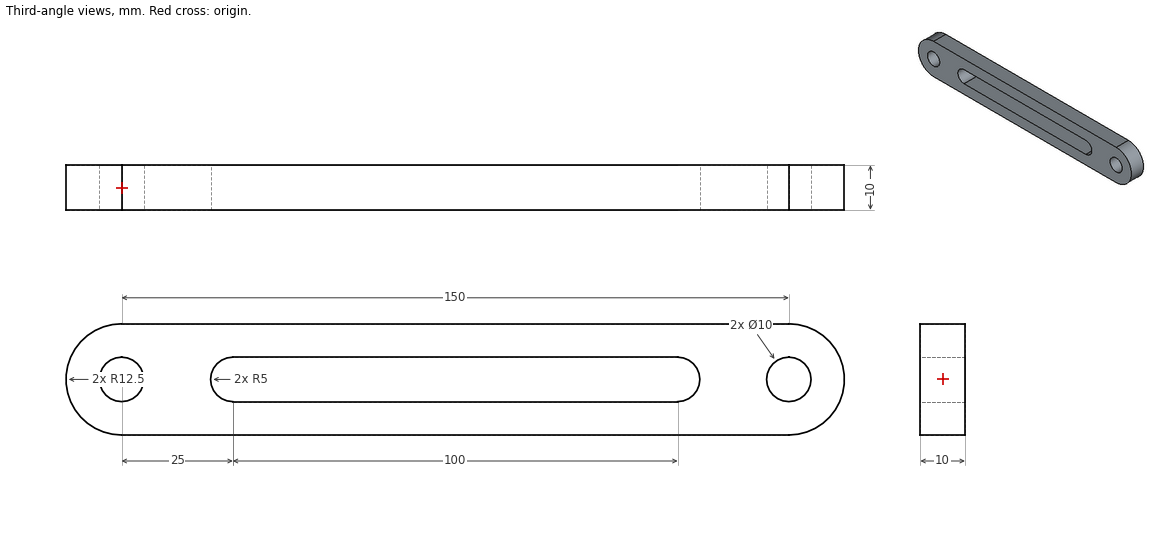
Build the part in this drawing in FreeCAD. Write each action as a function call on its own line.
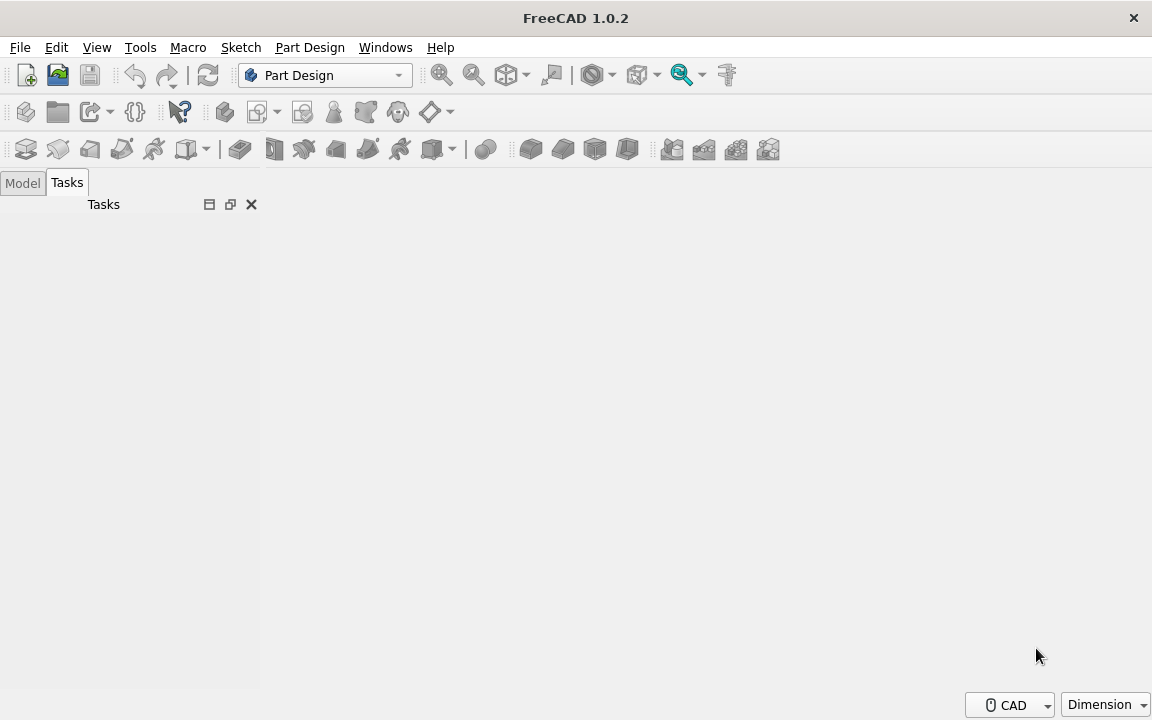
click(510, 112)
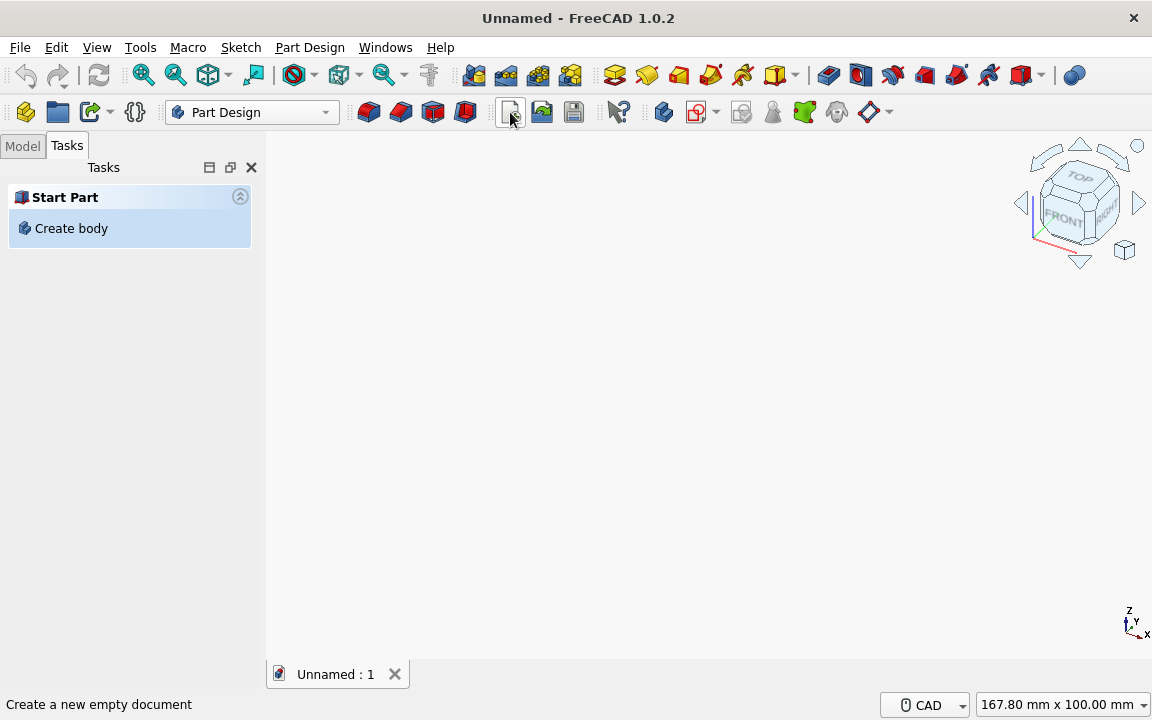
click(696, 112)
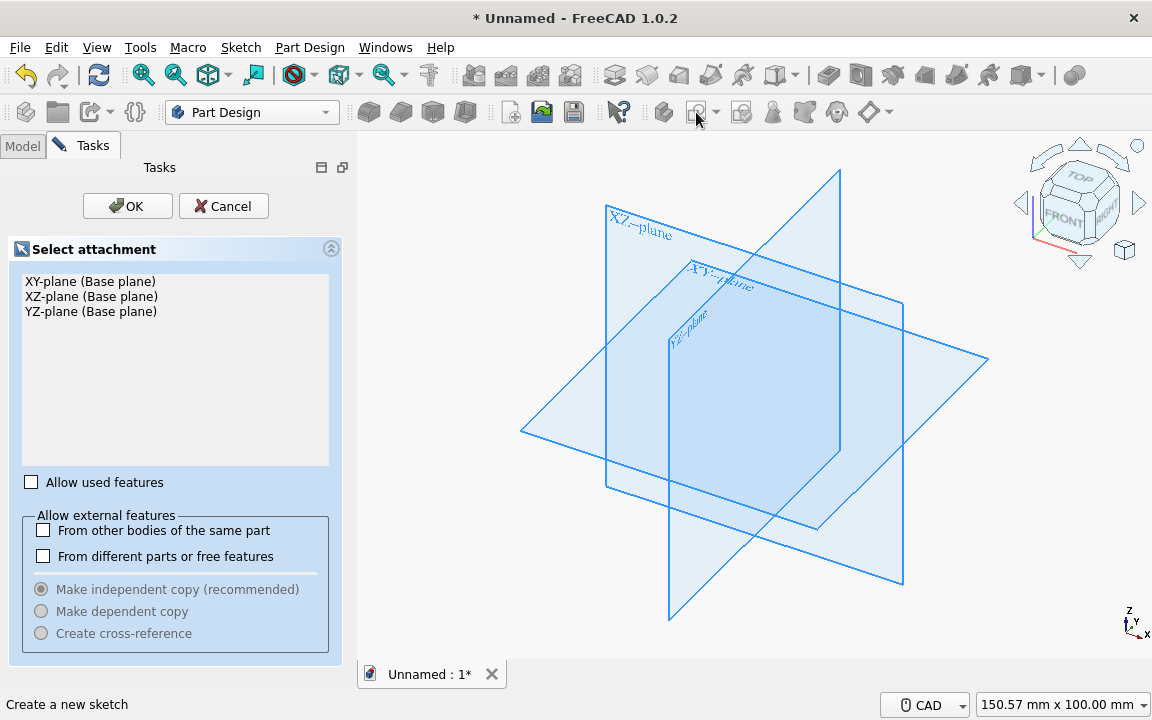
click(82, 296)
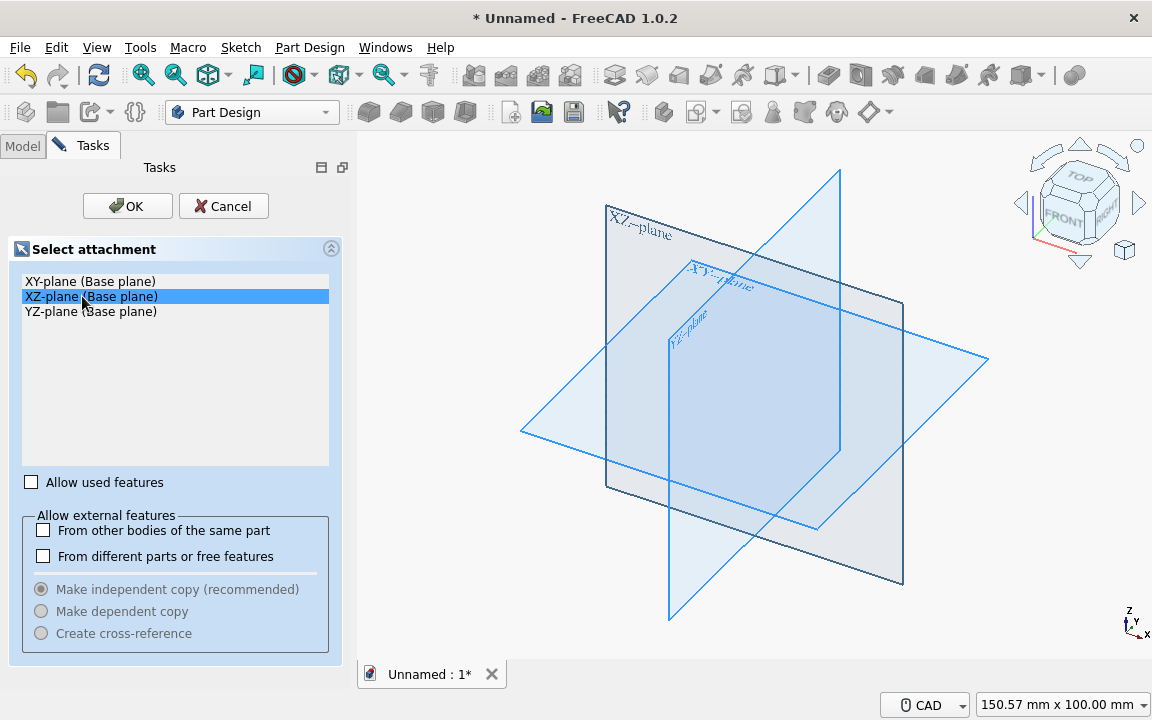
click(128, 206)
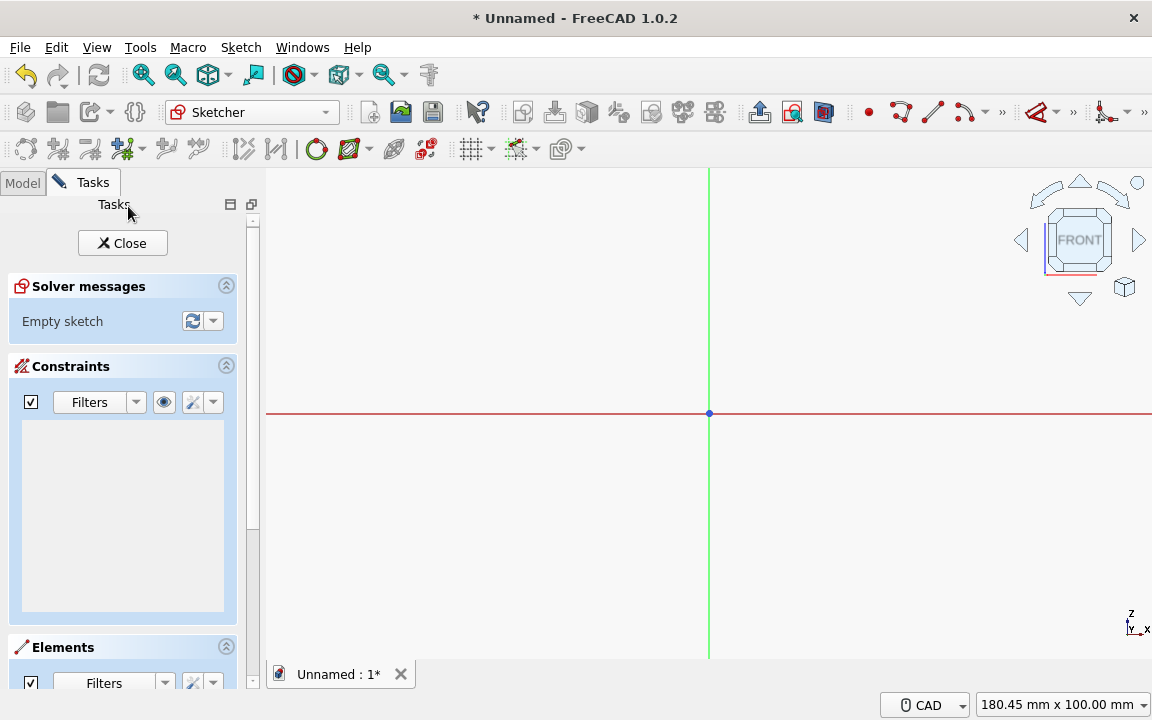
scroll(294, 414, down, 3)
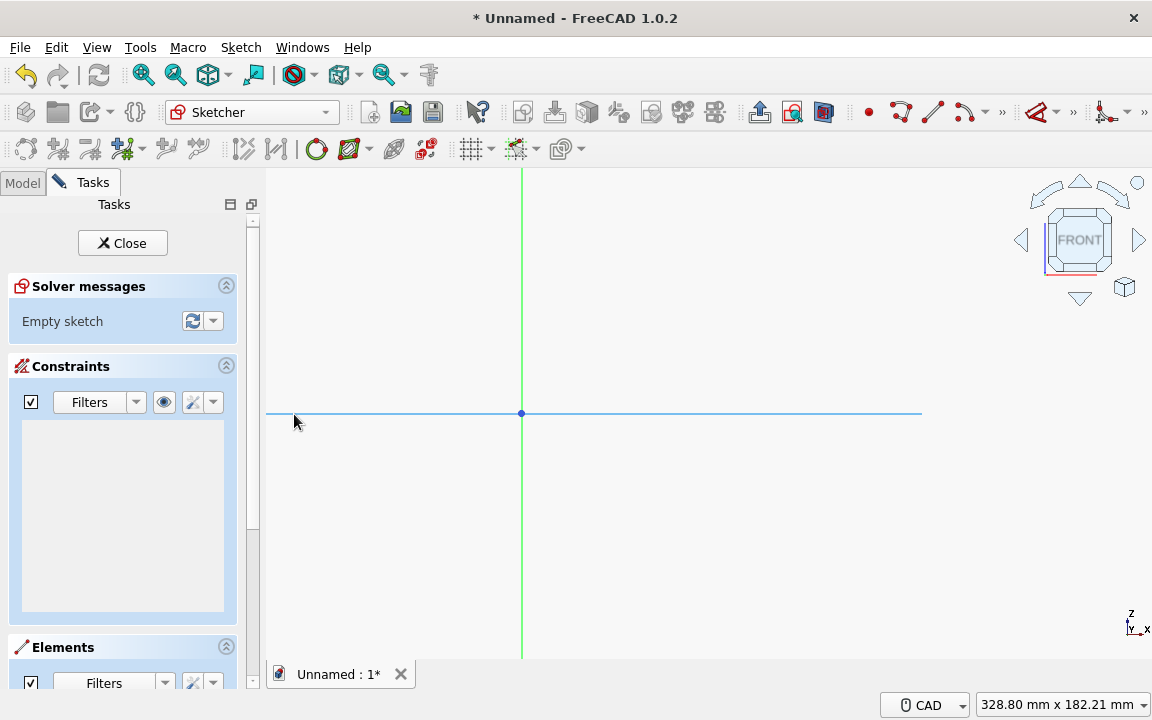
key(g)
key(s)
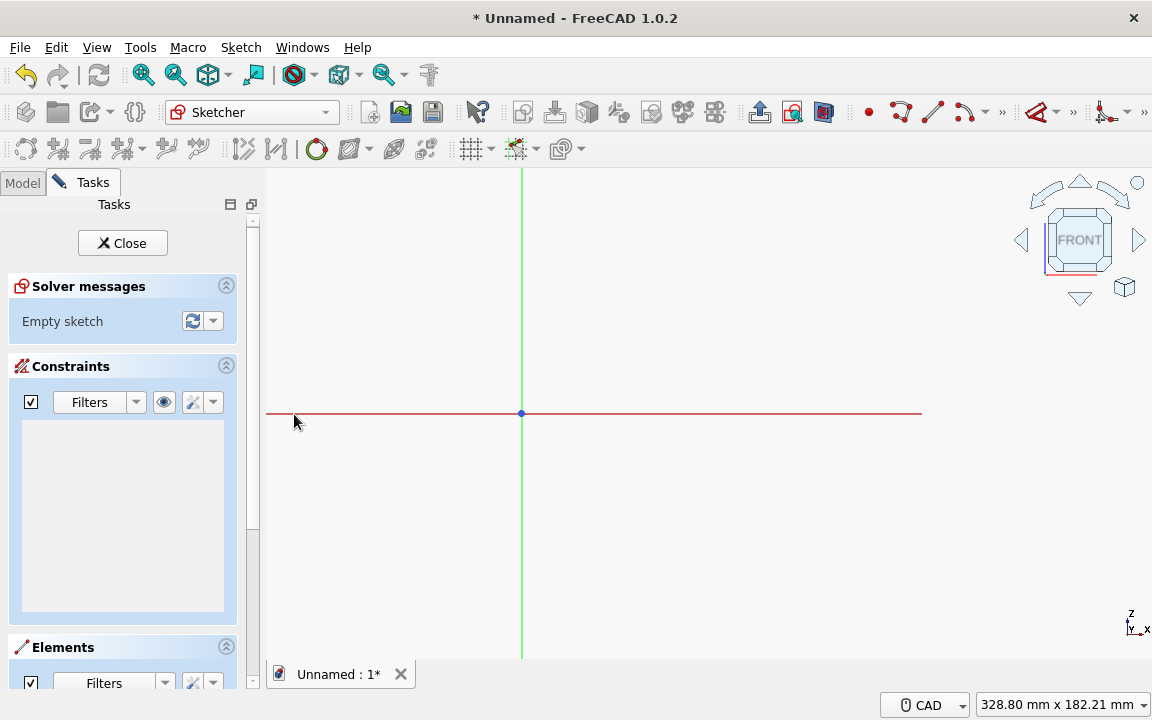
click(522, 414)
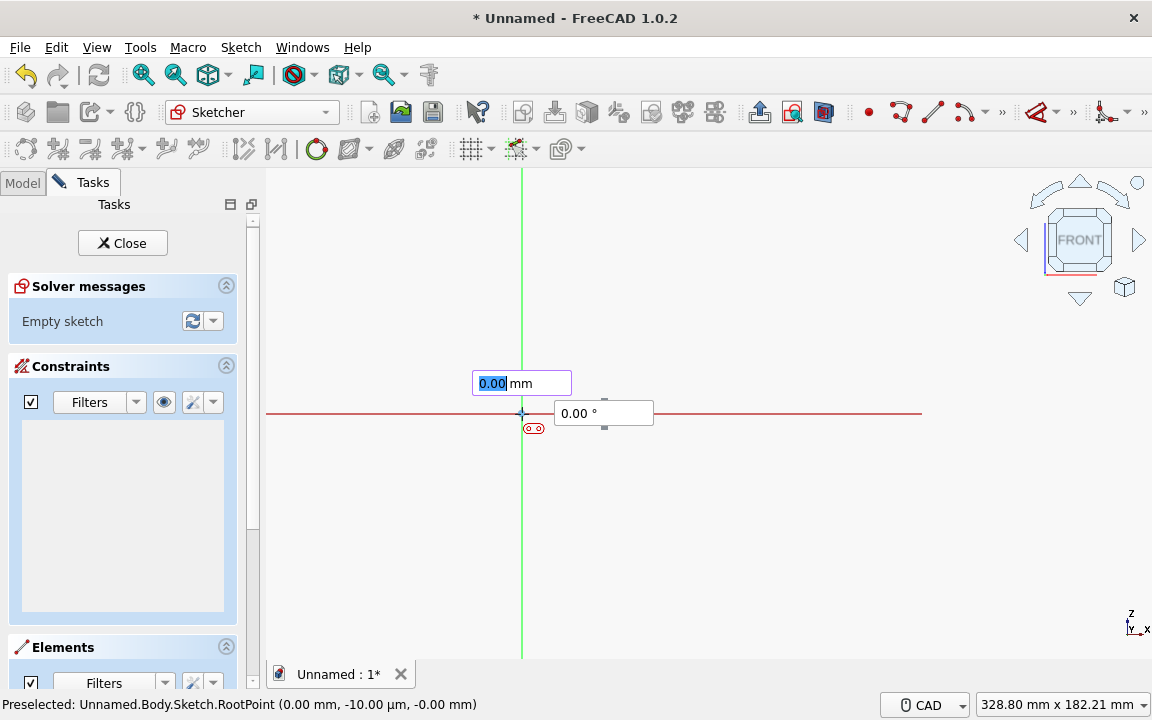
click(926, 405)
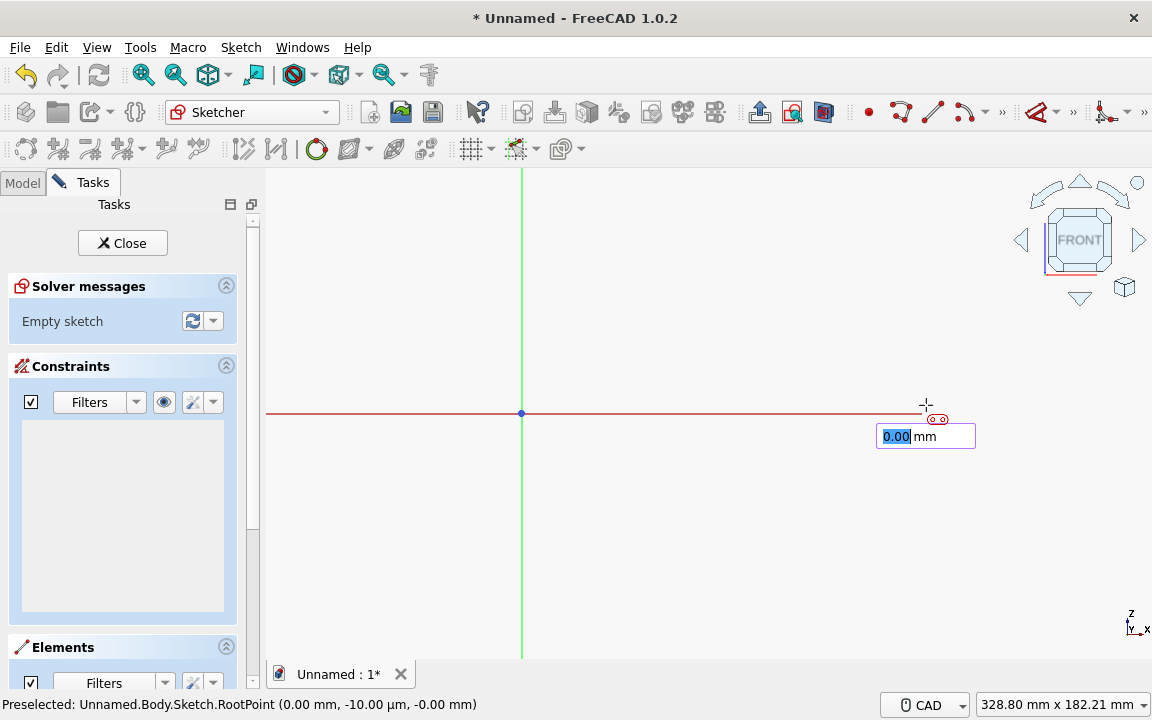
click(724, 448)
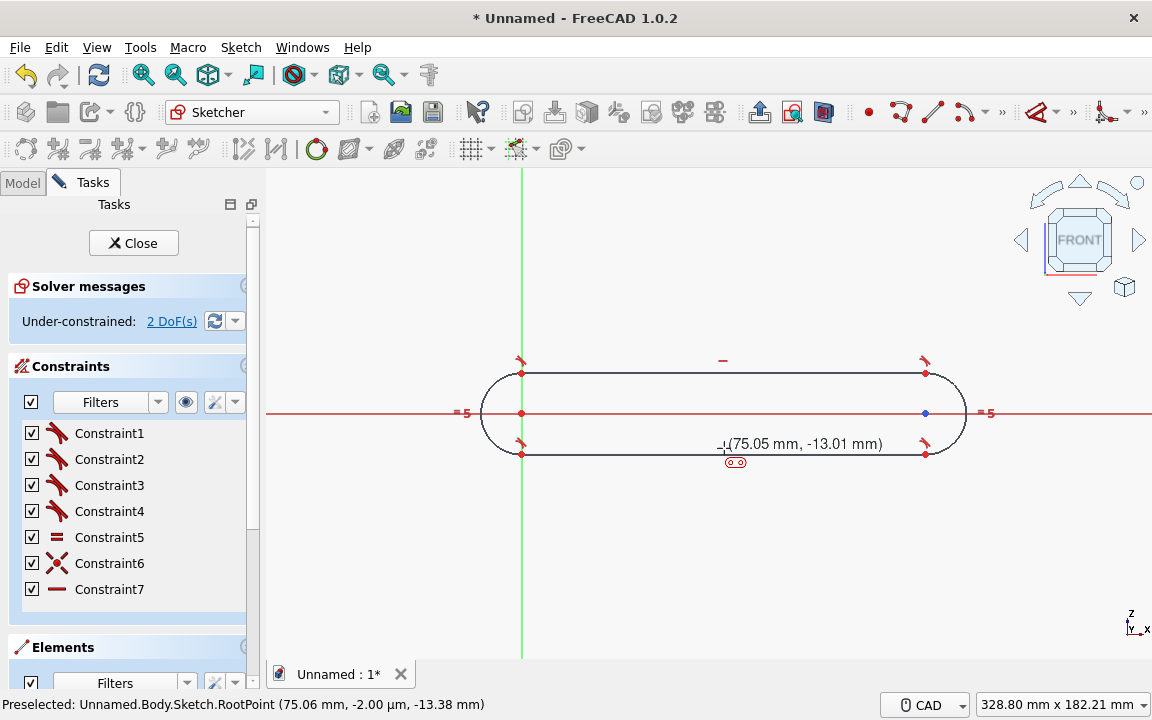
key(g)
key(c)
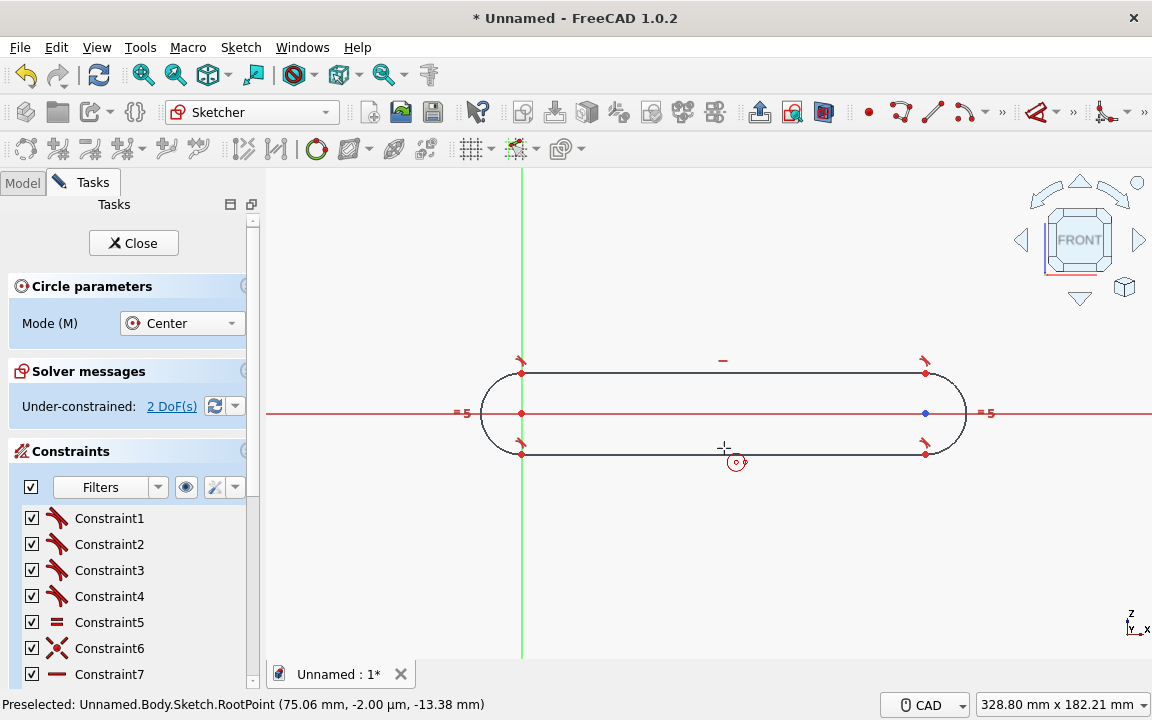
scroll(926, 414, up, 3)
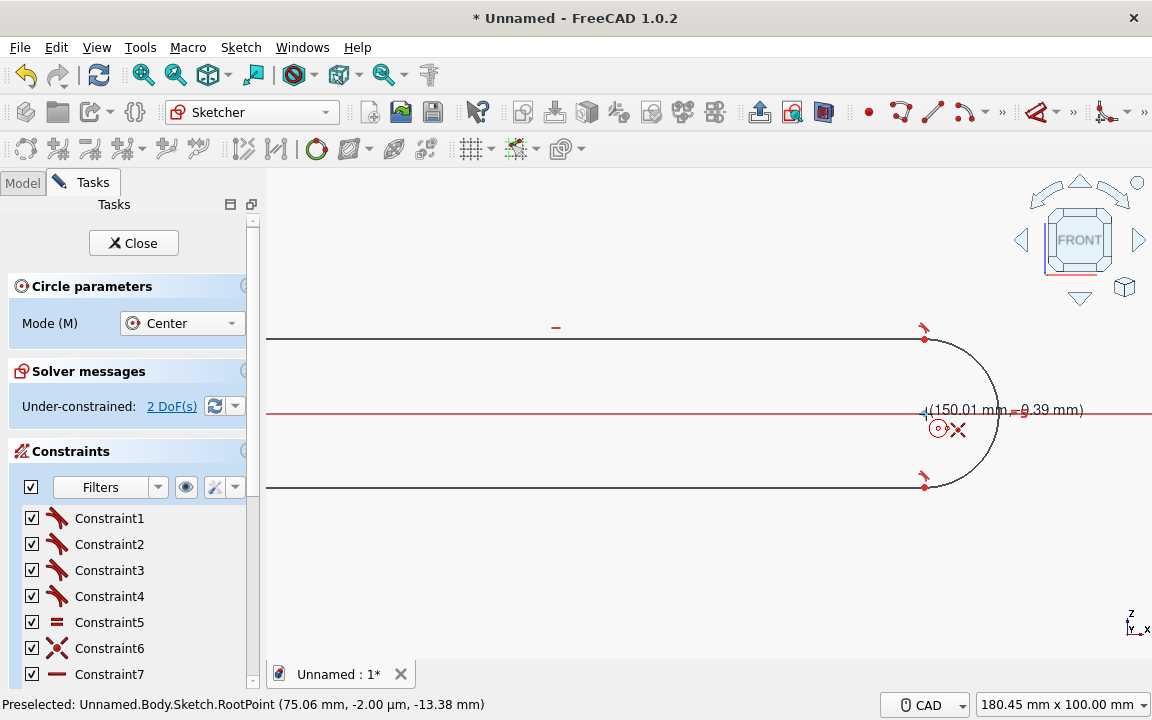
click(925, 397)
click(943, 396)